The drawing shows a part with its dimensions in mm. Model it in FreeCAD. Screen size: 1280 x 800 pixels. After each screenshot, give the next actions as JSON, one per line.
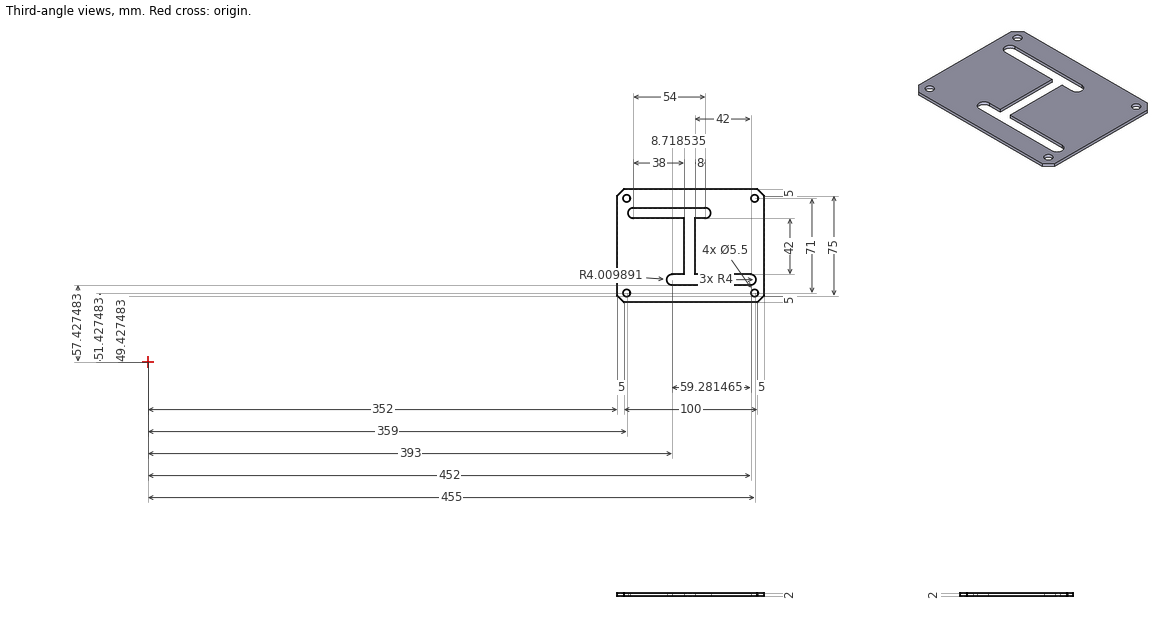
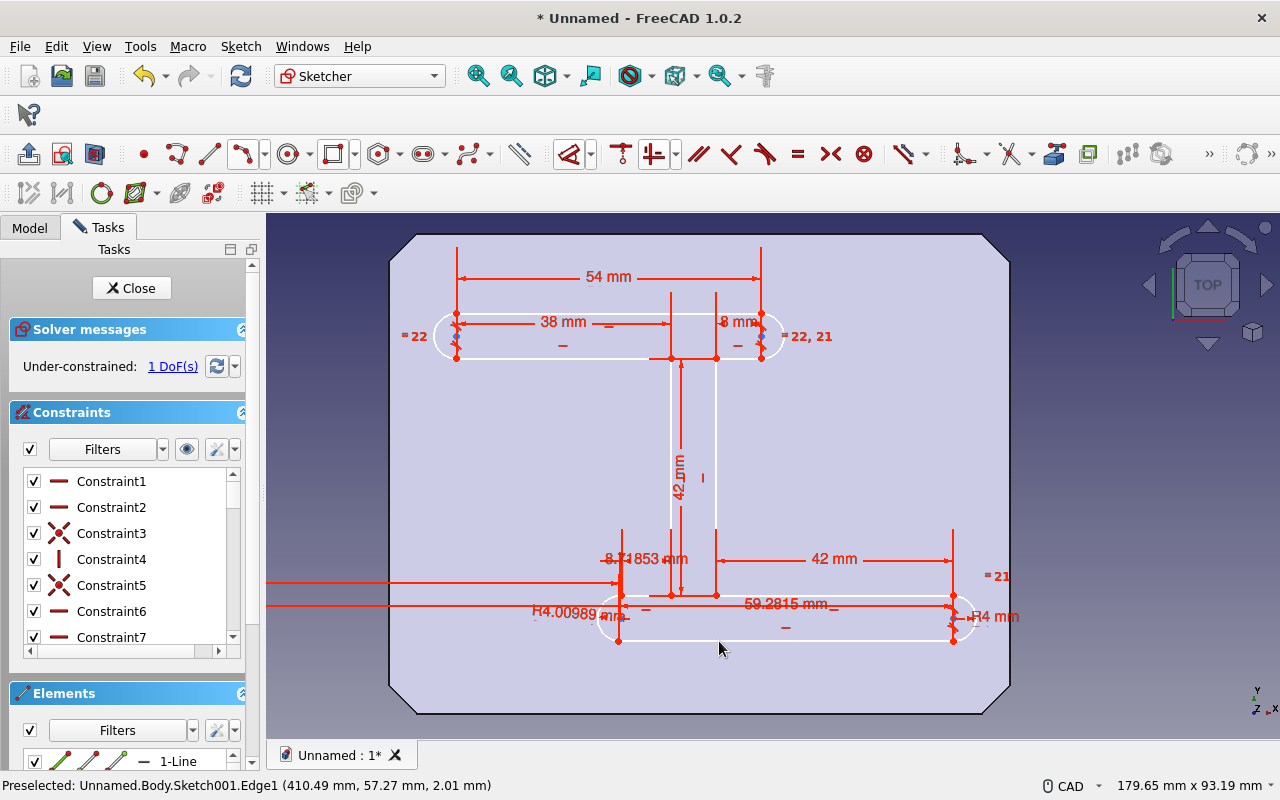
{"action": "left_click", "coordinate": [619, 641]}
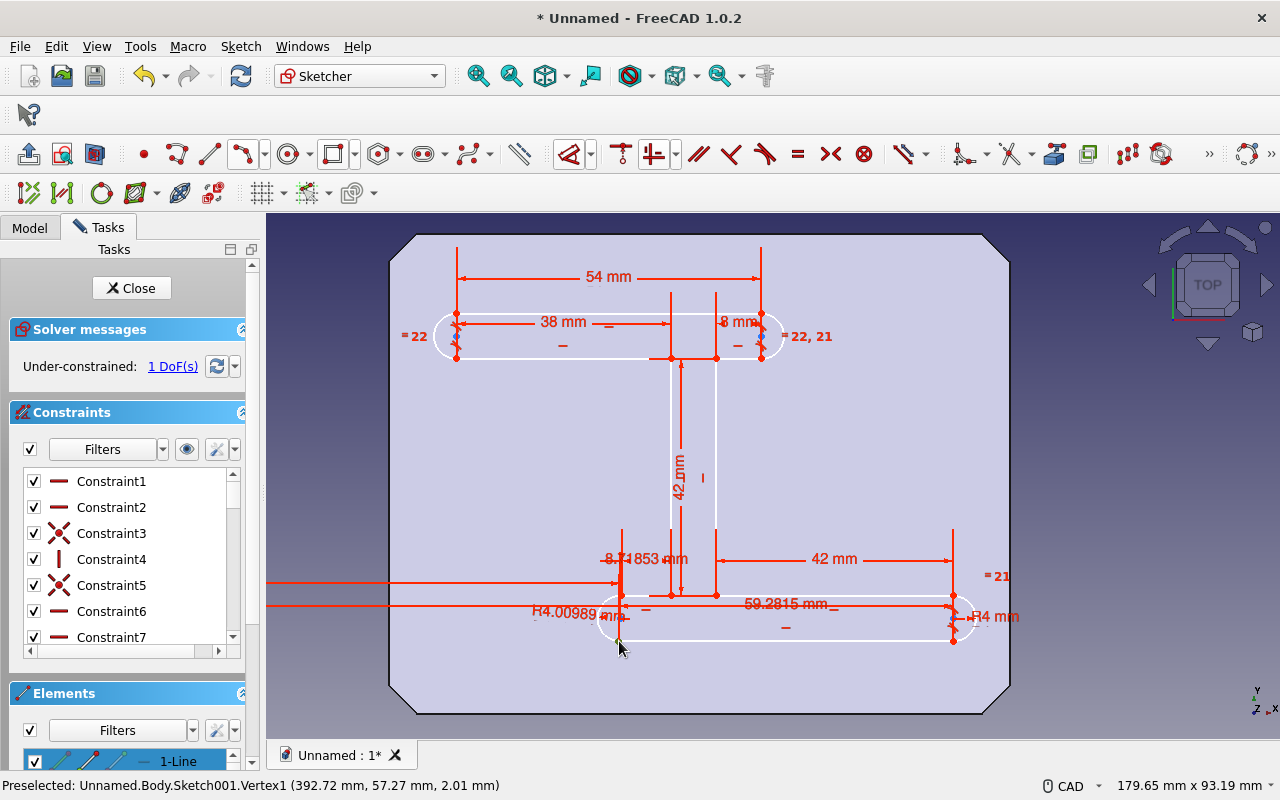
{"action": "key", "text": "i"}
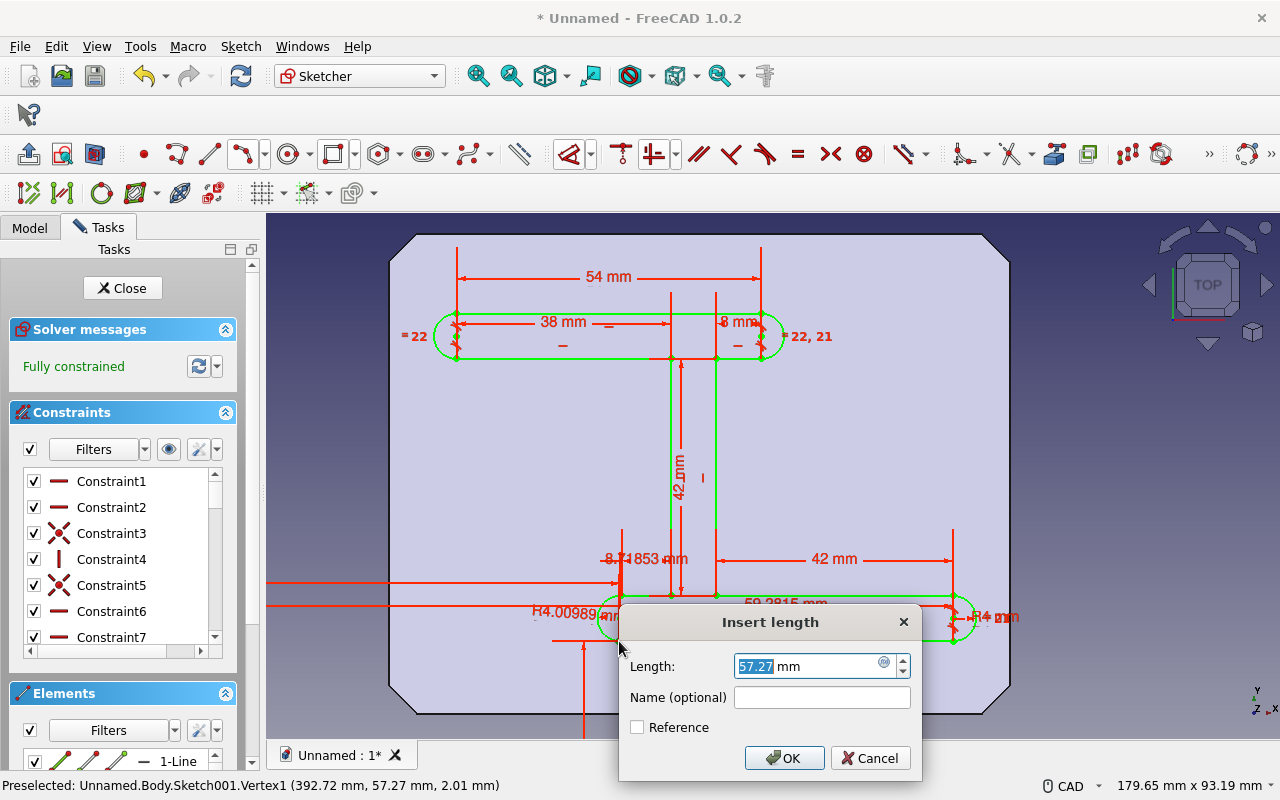
{"action": "type", "text": "57.427483"}
{"action": "key", "text": "Return"}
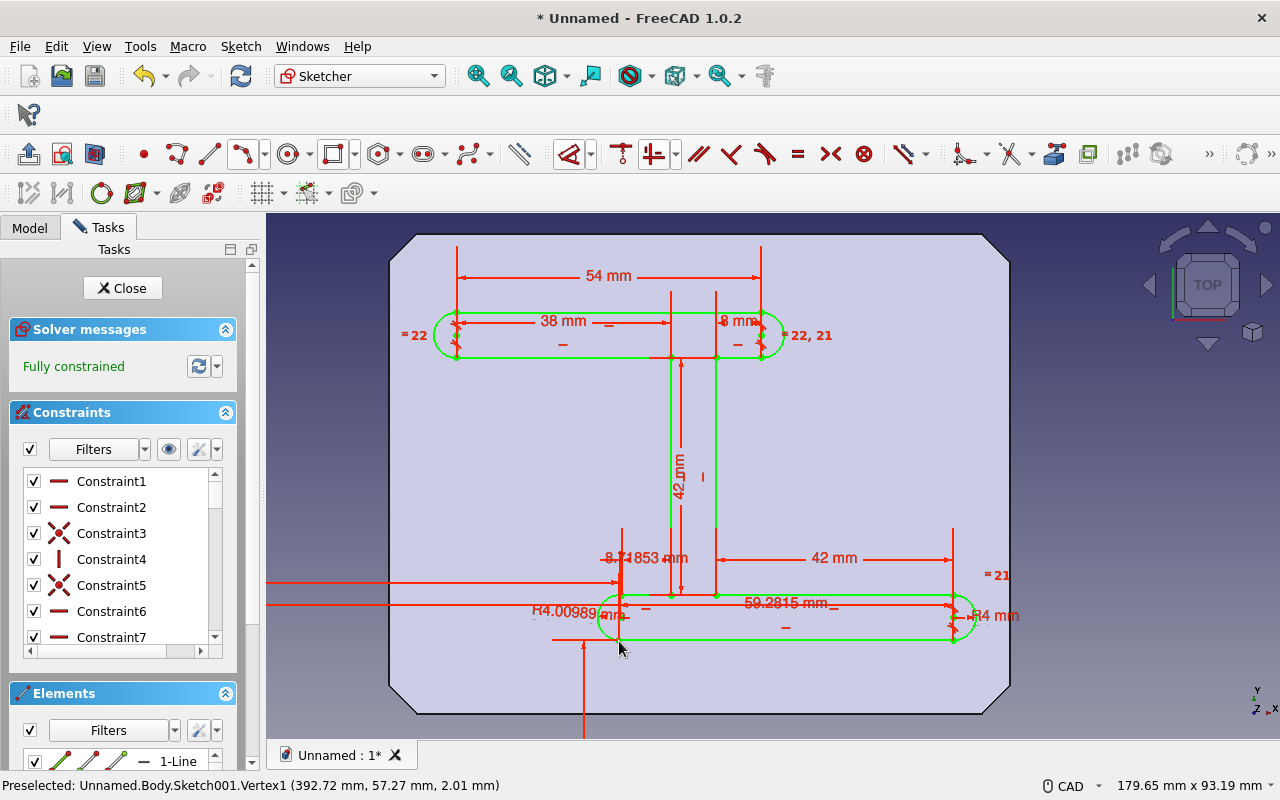
{"action": "left_click", "coordinate": [123, 288]}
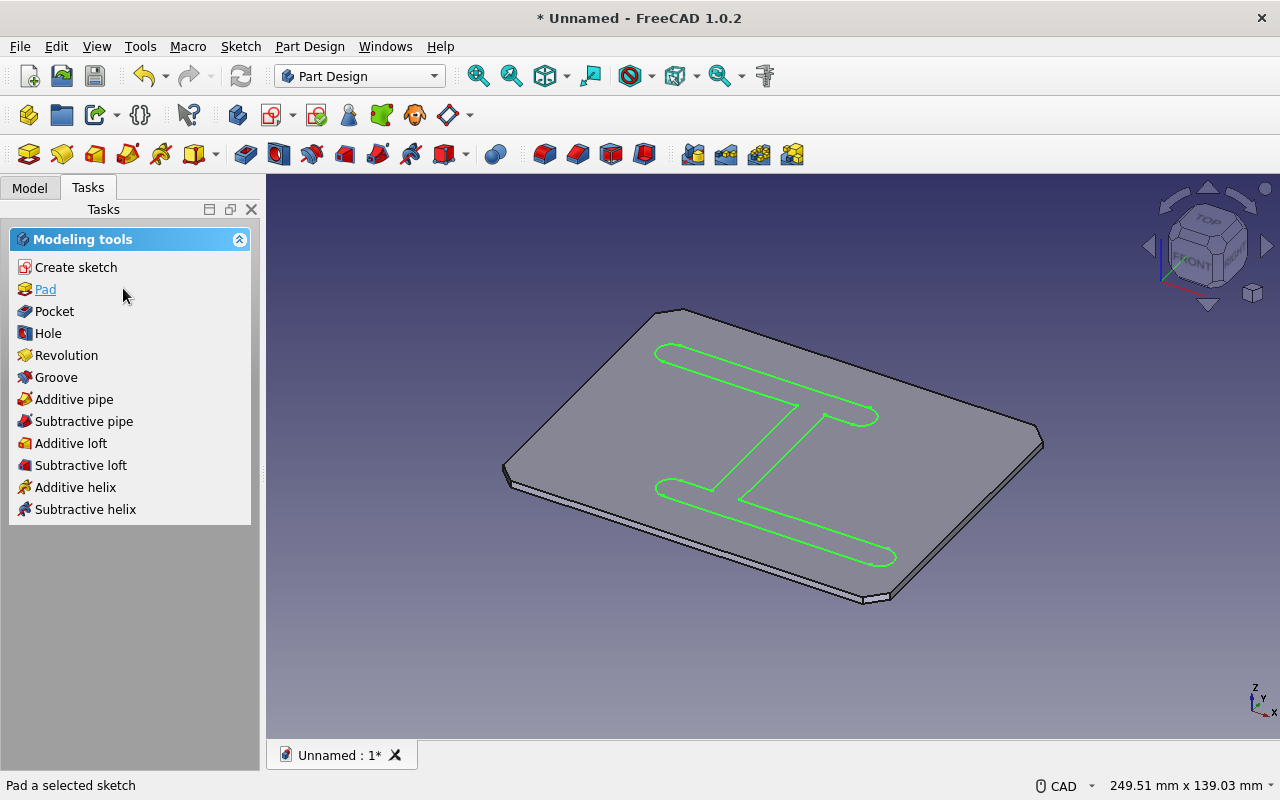
{"action": "left_click", "coordinate": [246, 154]}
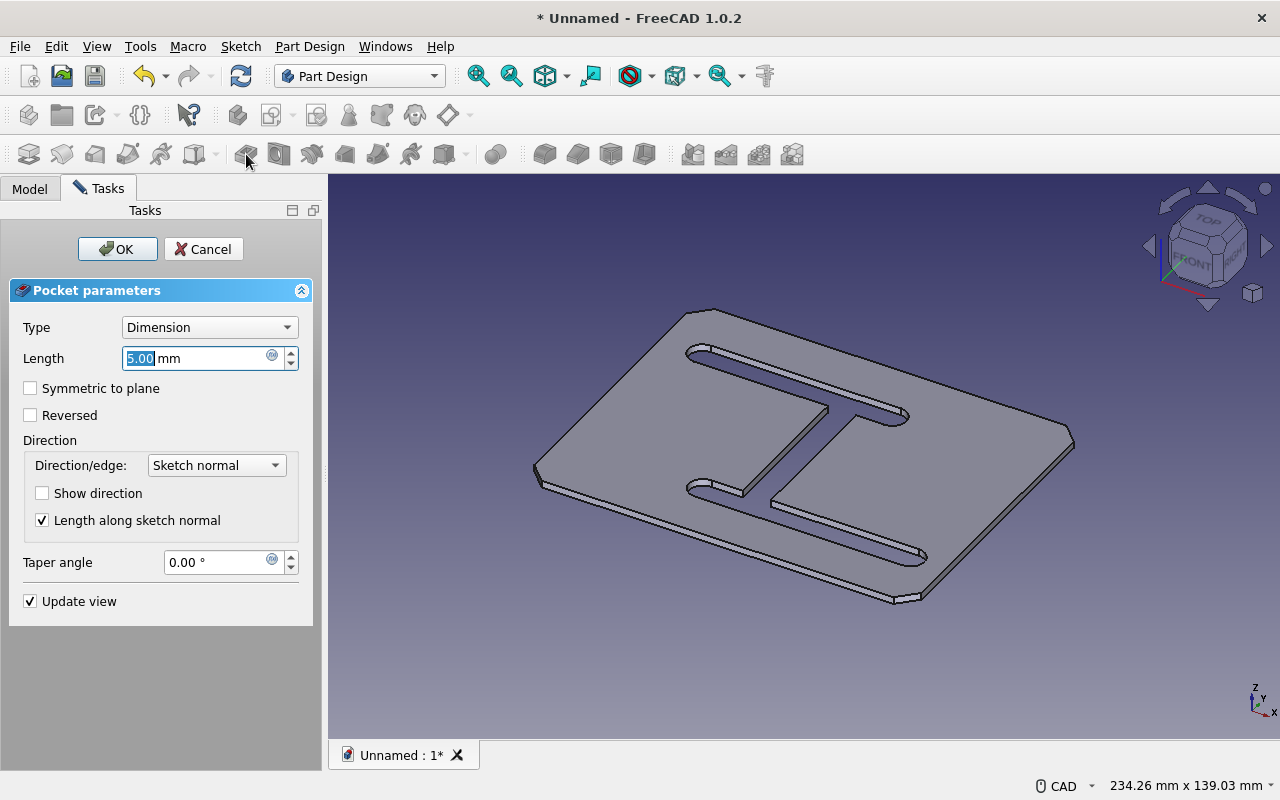
{"action": "type", "text": "2"}
{"action": "key", "text": "Tab"}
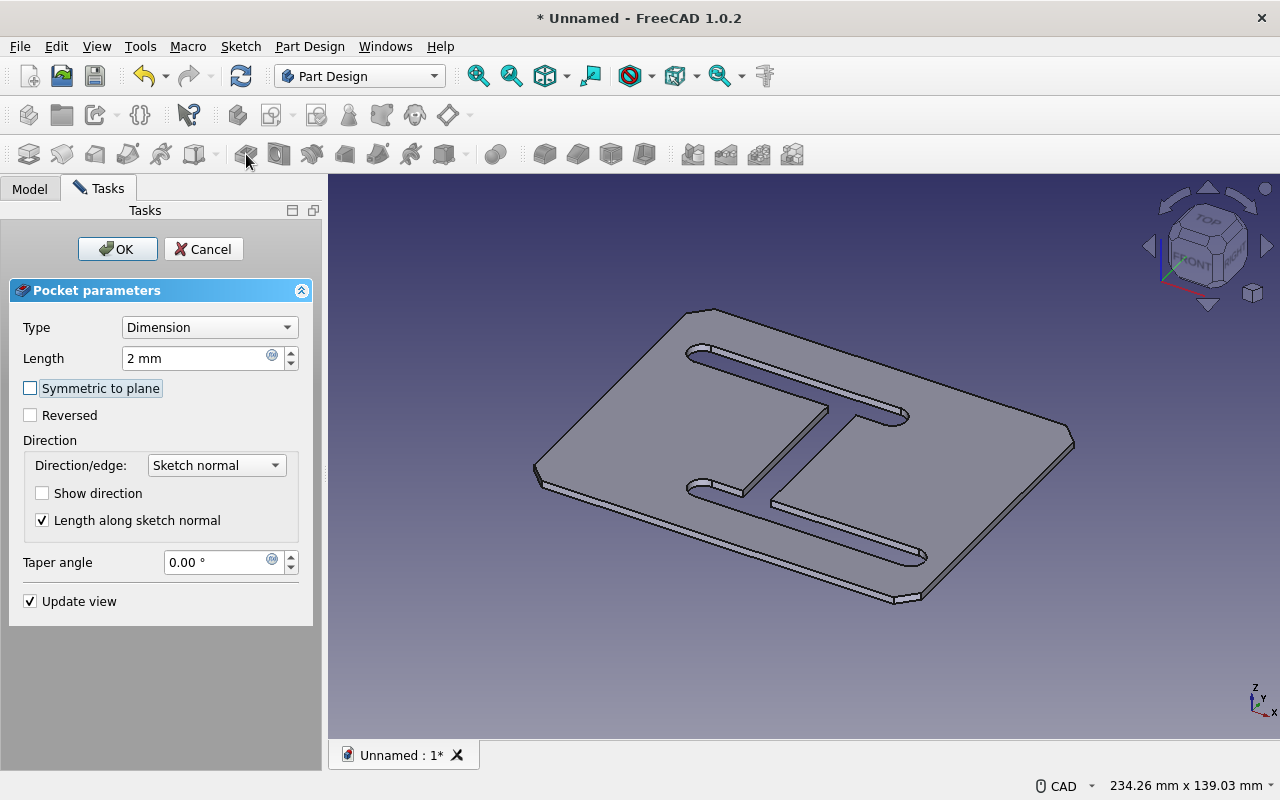
{"action": "left_click", "coordinate": [118, 249]}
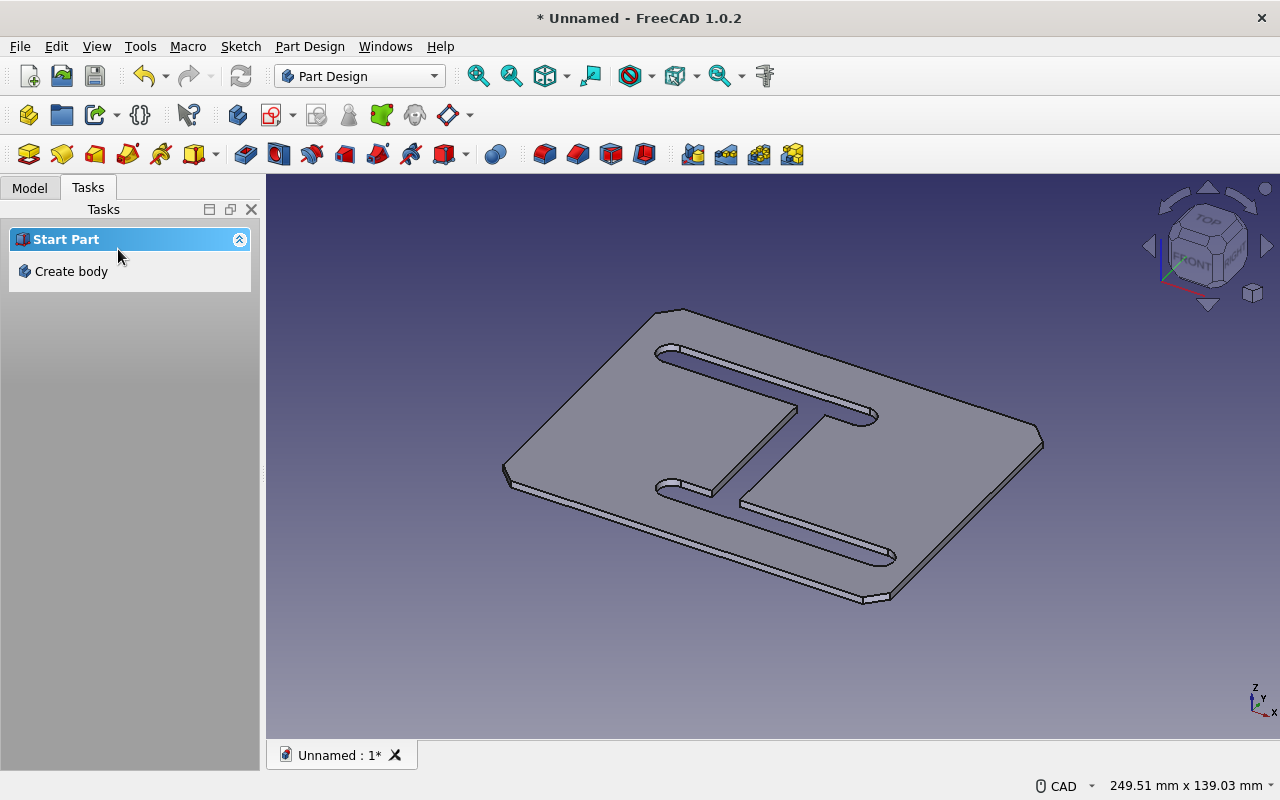
{"action": "left_click", "coordinate": [884, 489]}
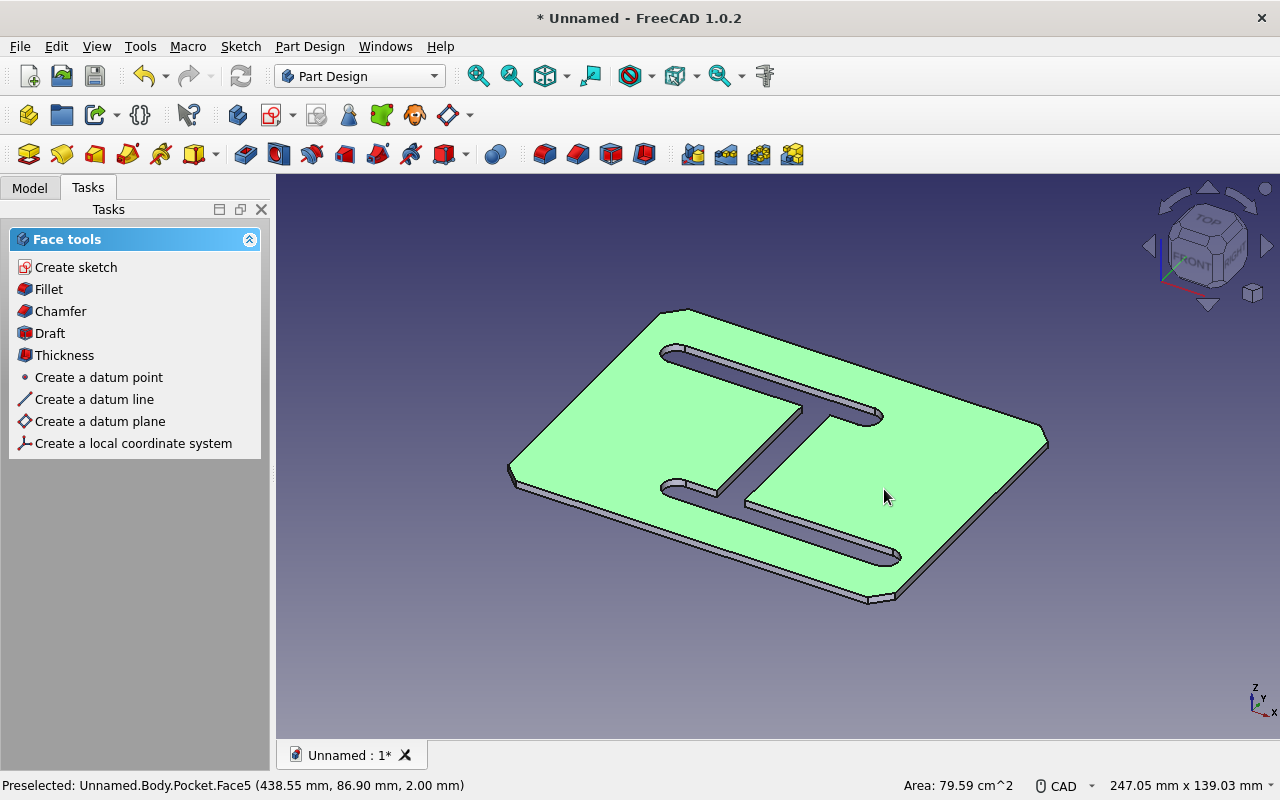
{"action": "left_click", "coordinate": [270, 116]}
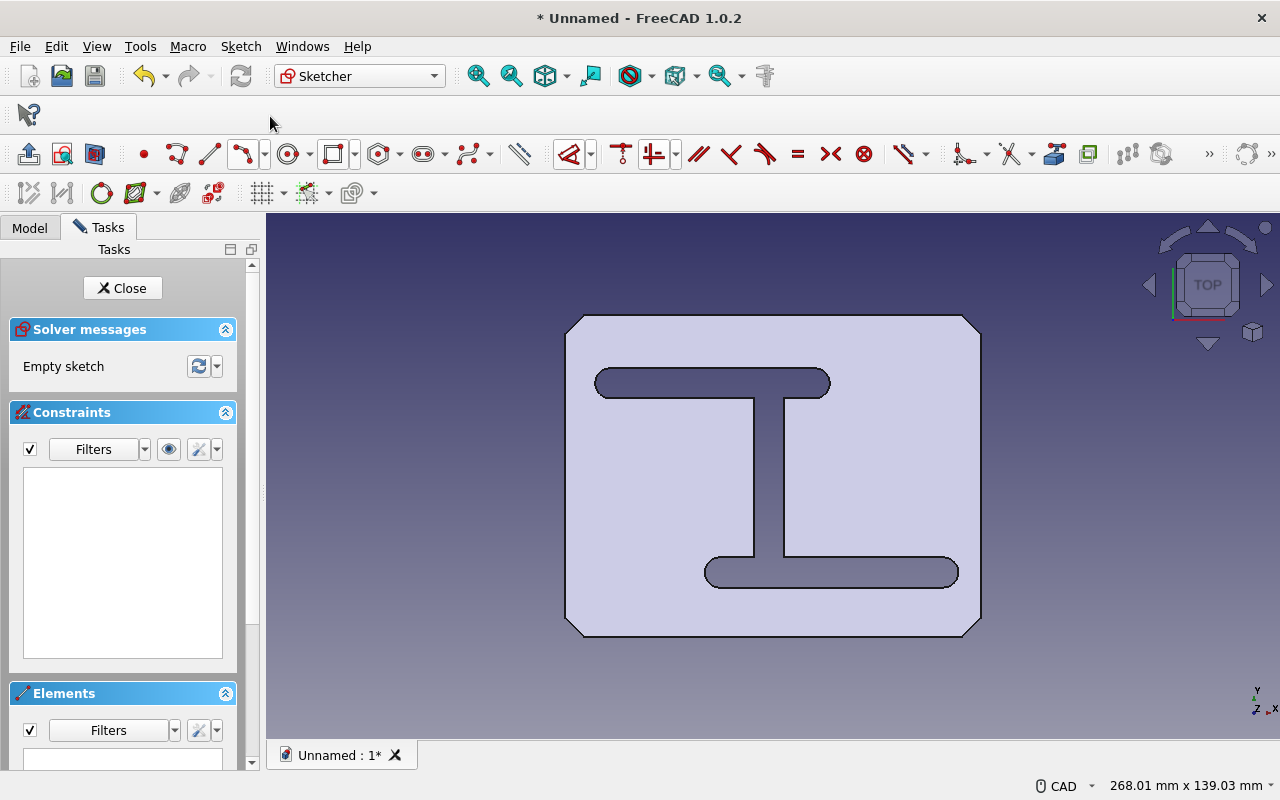
{"action": "key", "text": "g c"}